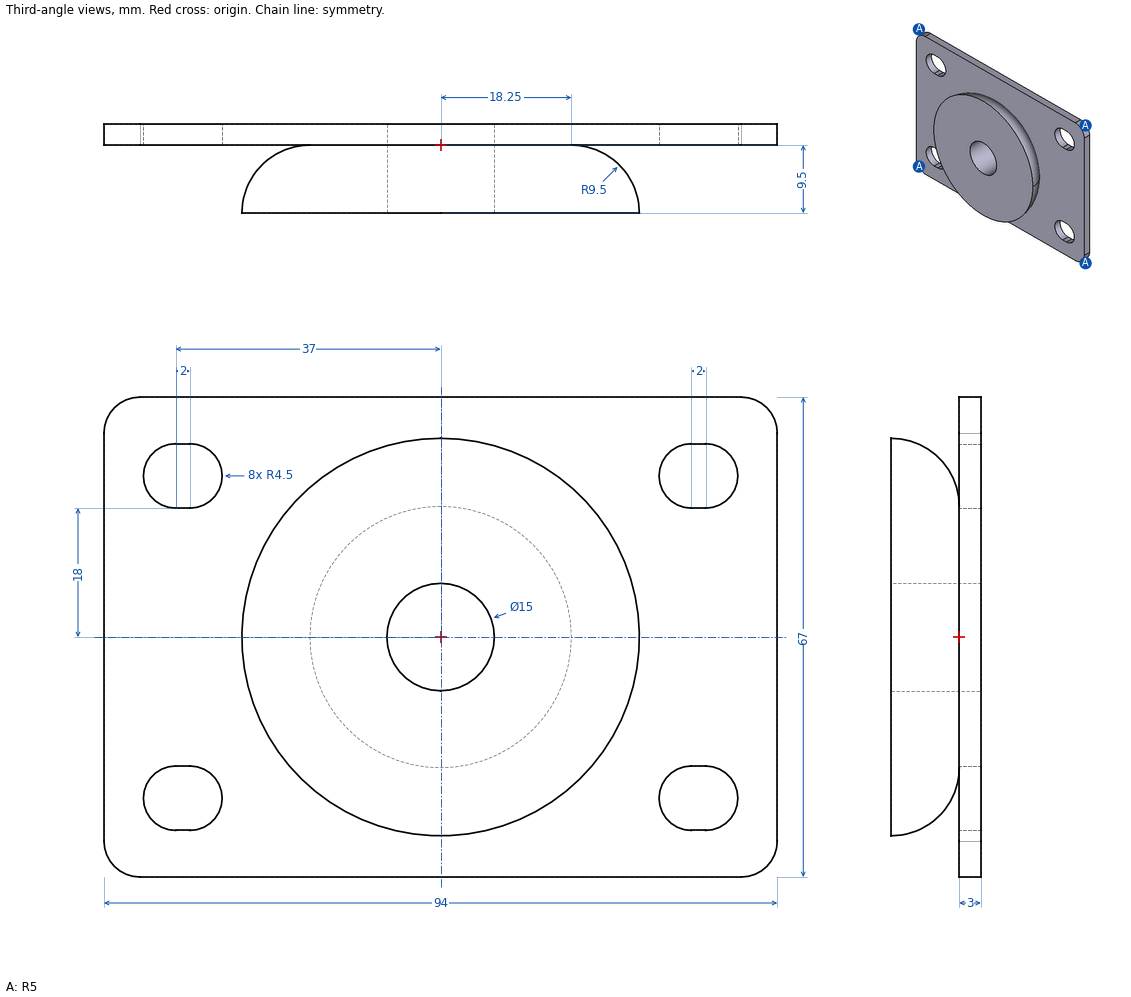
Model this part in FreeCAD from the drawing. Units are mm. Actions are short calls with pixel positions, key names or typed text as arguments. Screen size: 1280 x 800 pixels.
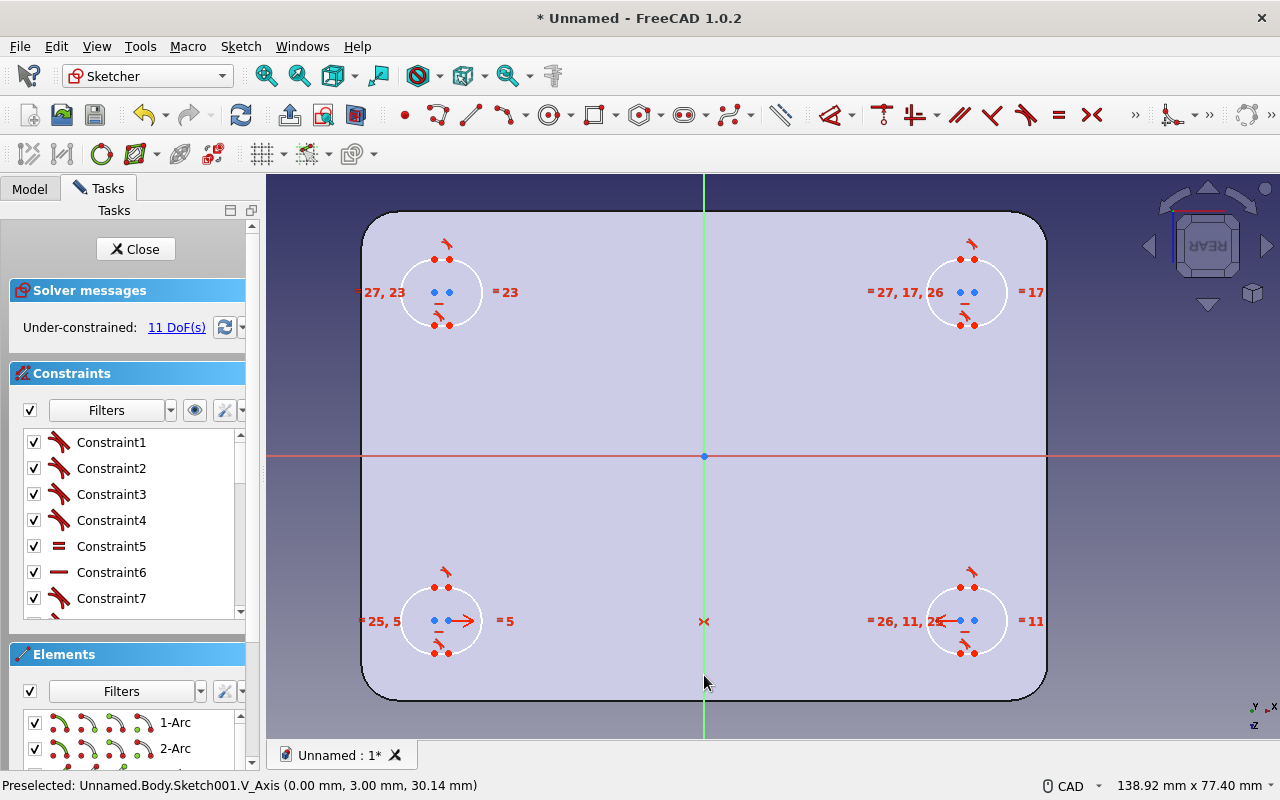
click(960, 621)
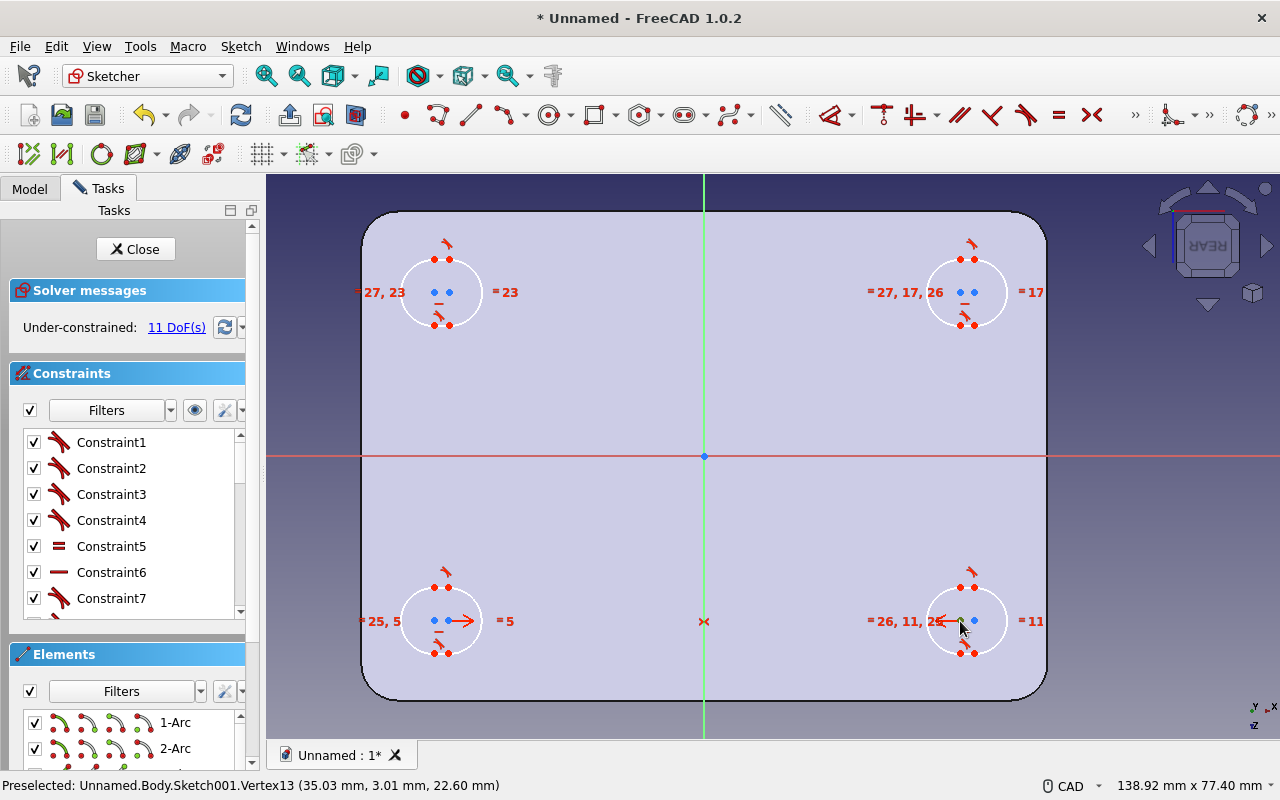
click(960, 293)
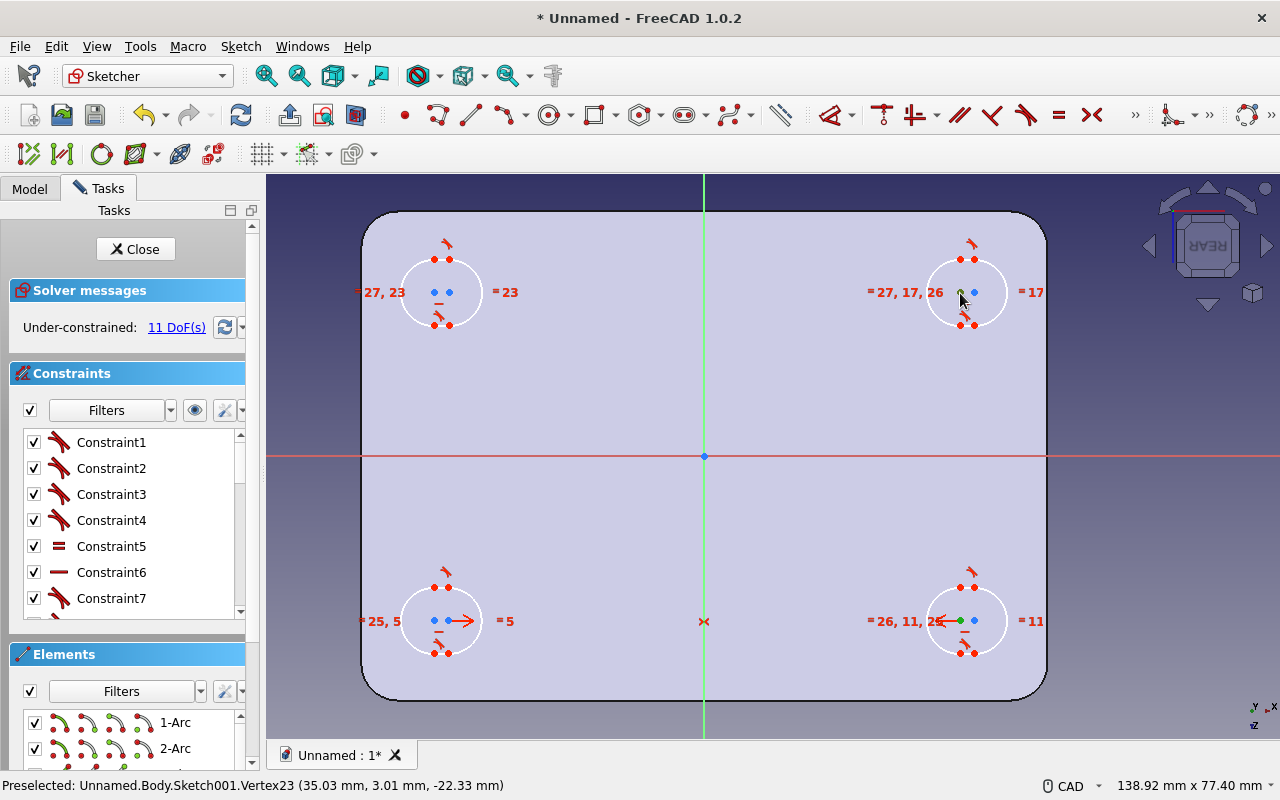
click(353, 456)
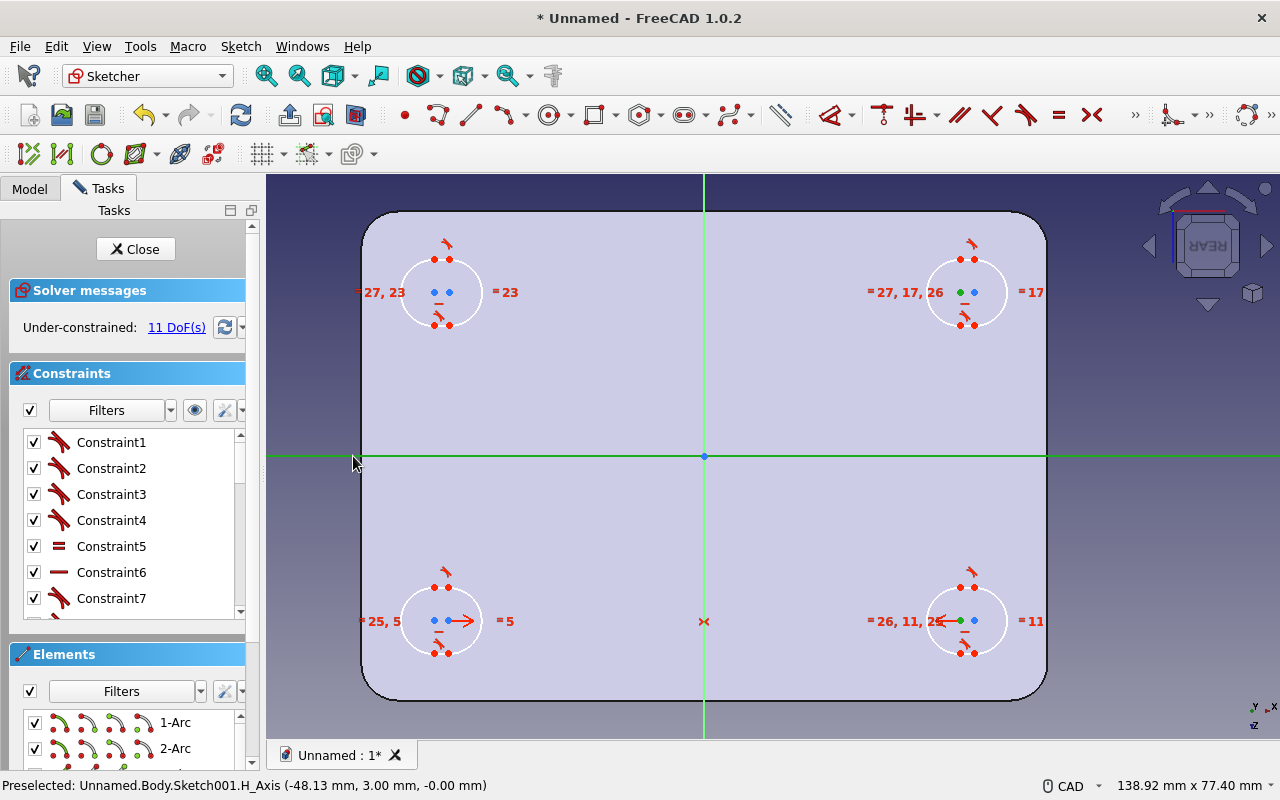
key(s)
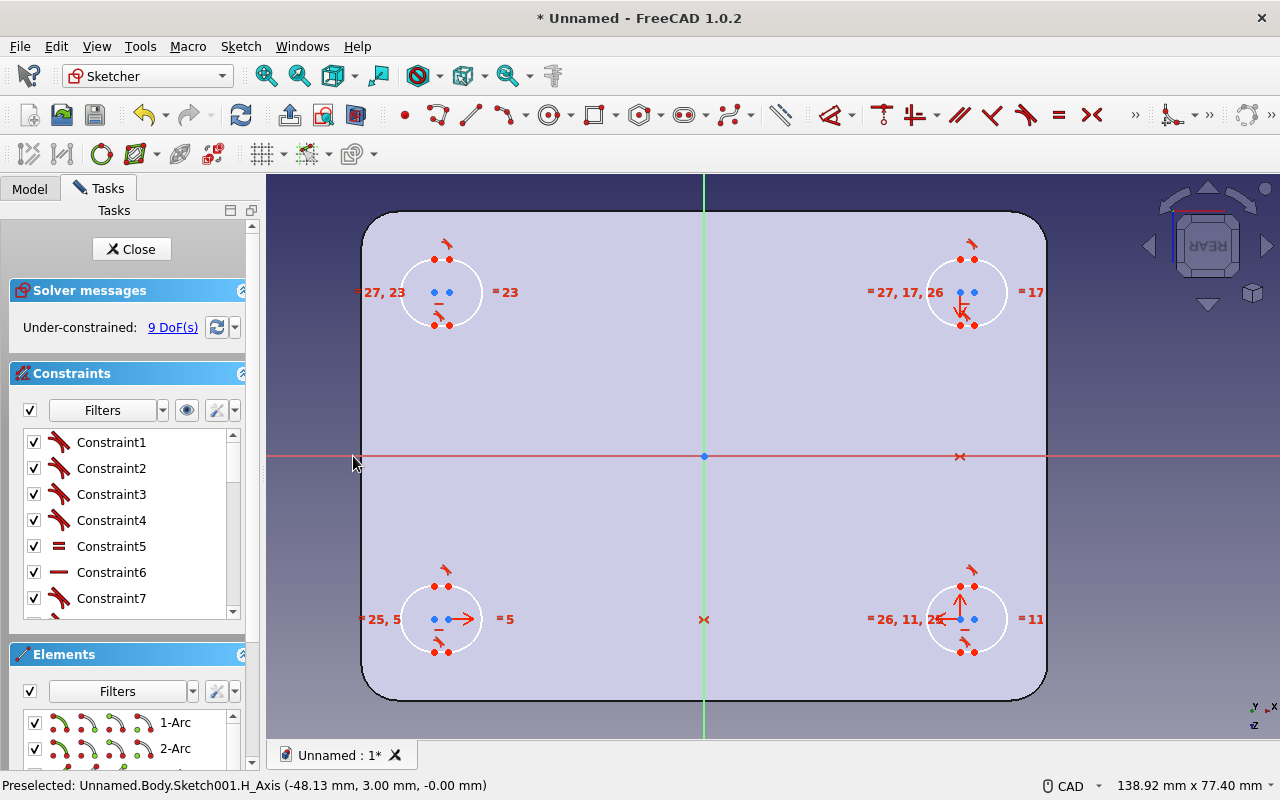
click(434, 619)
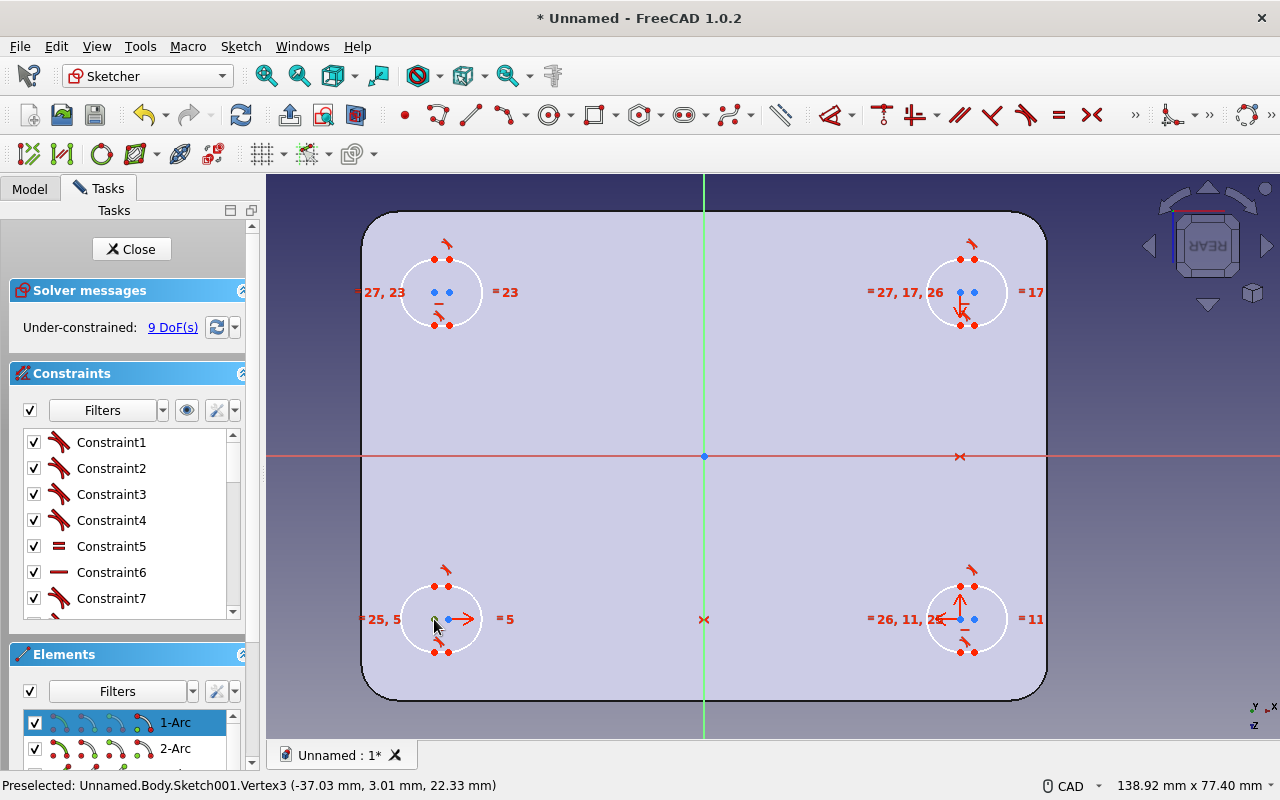
click(434, 293)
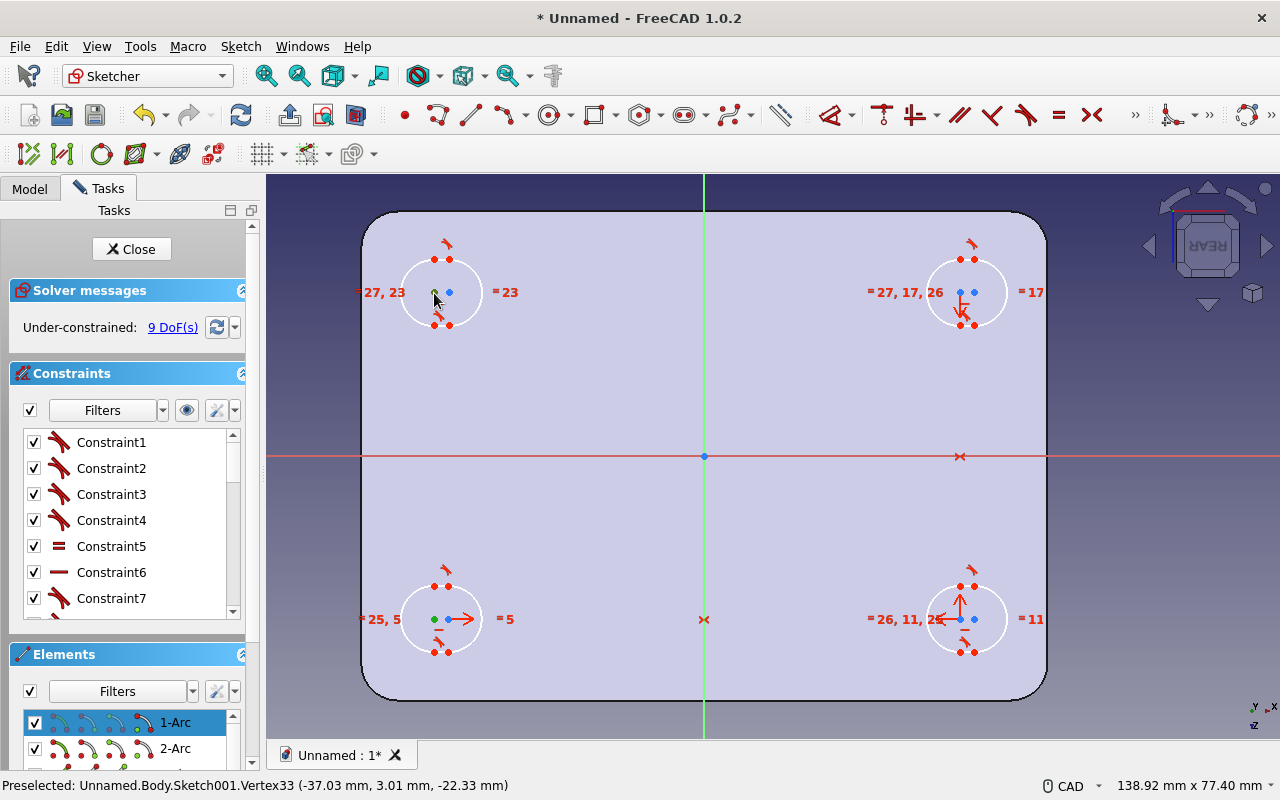
click(353, 456)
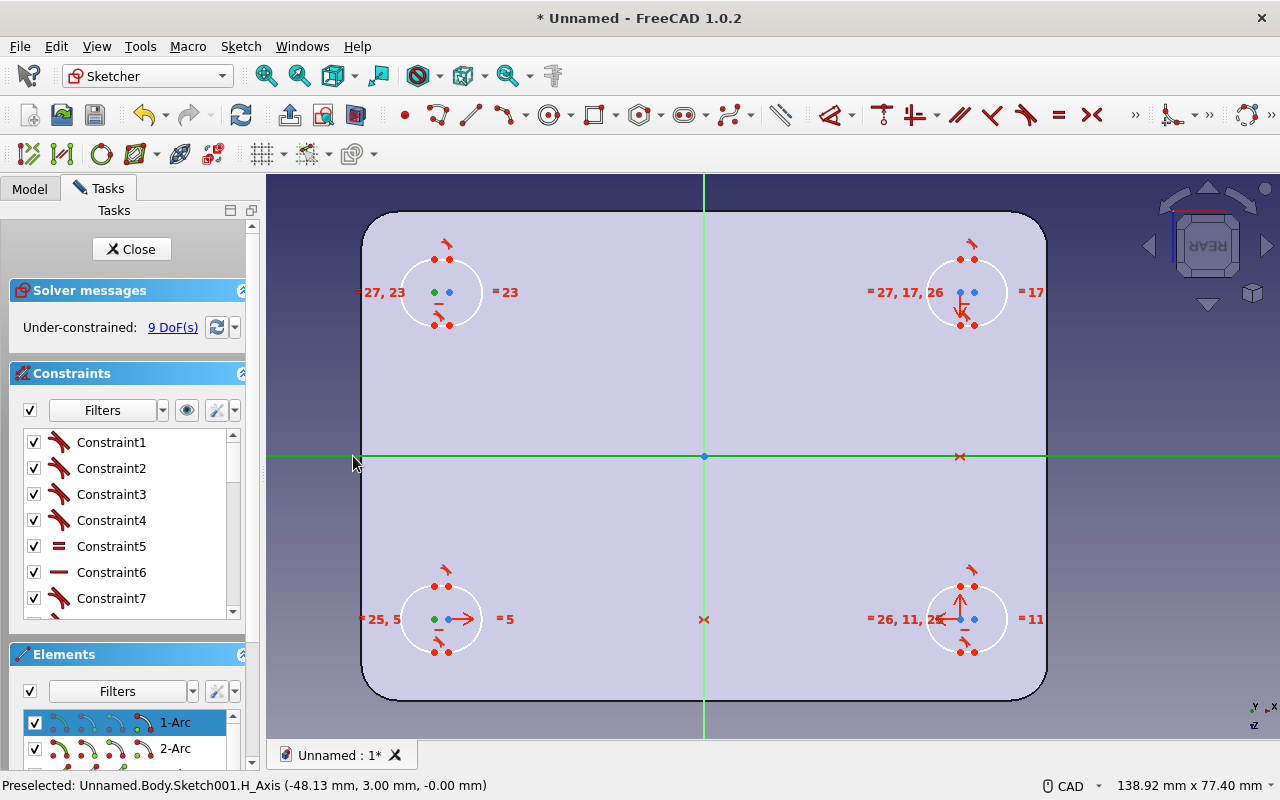
key(s)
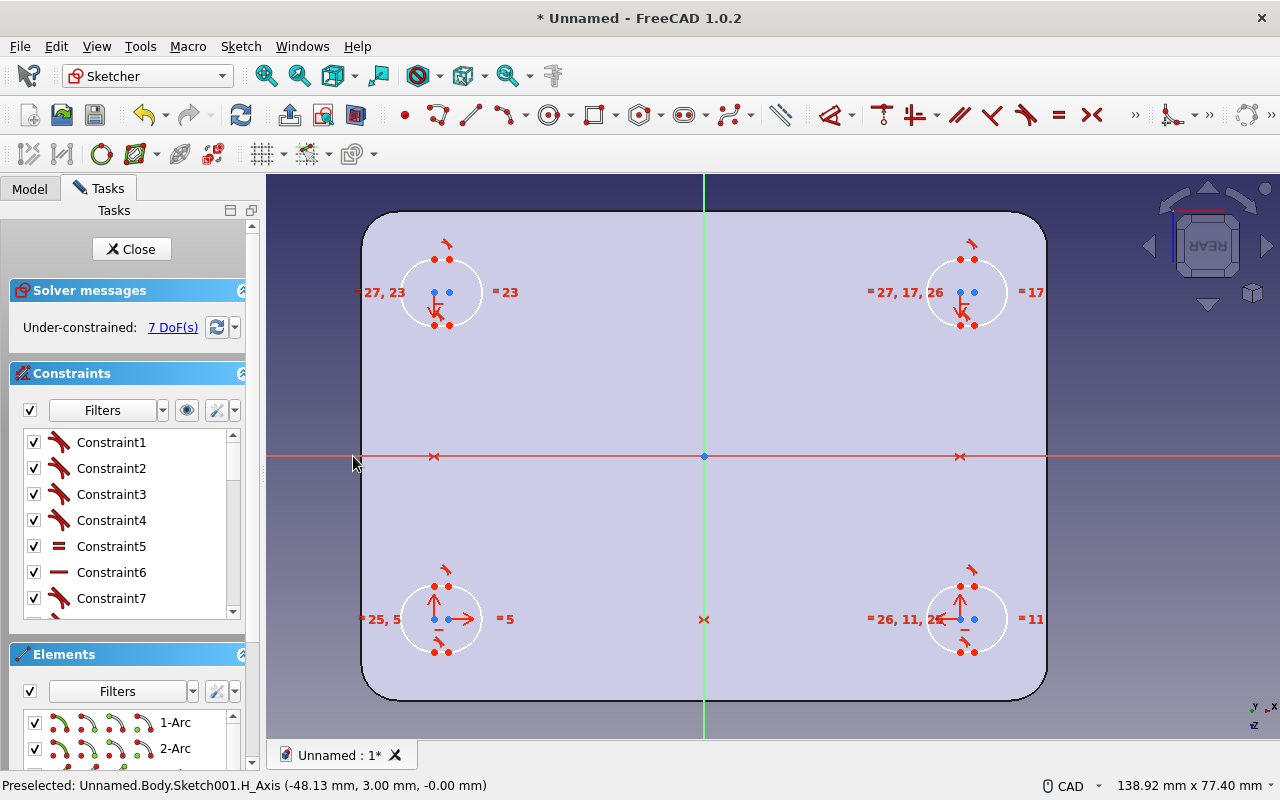
key(d)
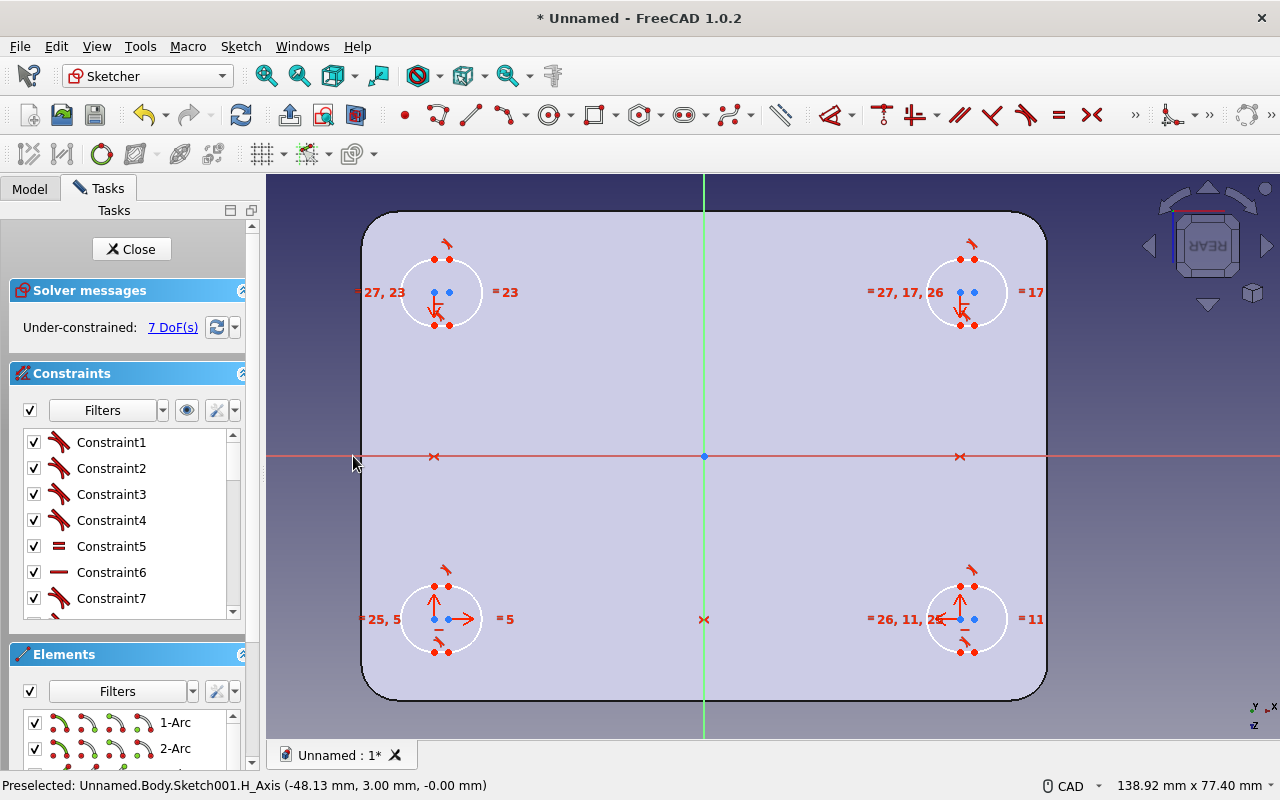
click(407, 600)
click(381, 582)